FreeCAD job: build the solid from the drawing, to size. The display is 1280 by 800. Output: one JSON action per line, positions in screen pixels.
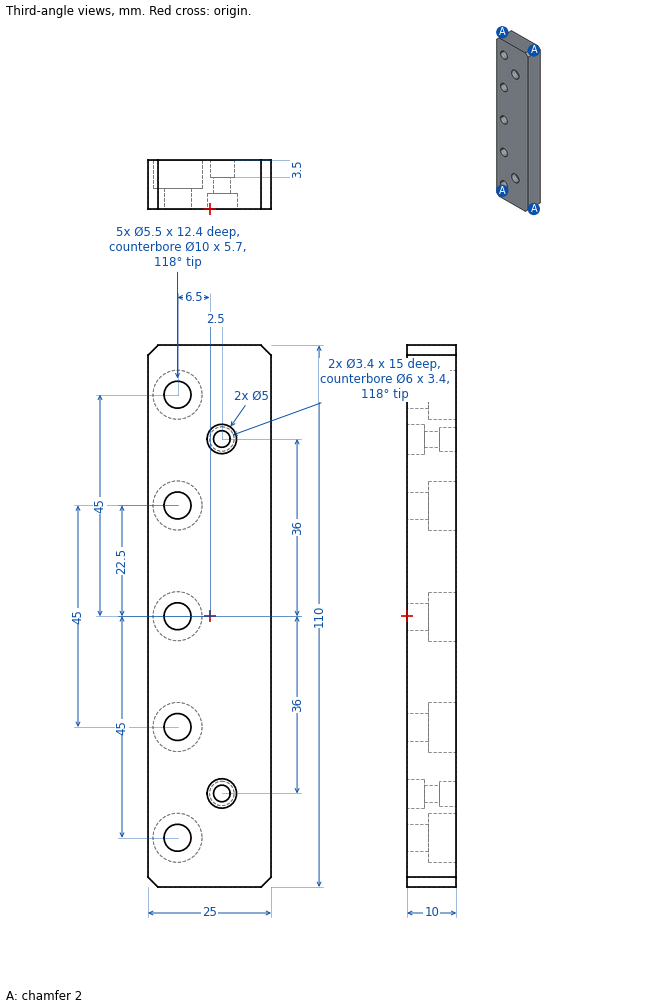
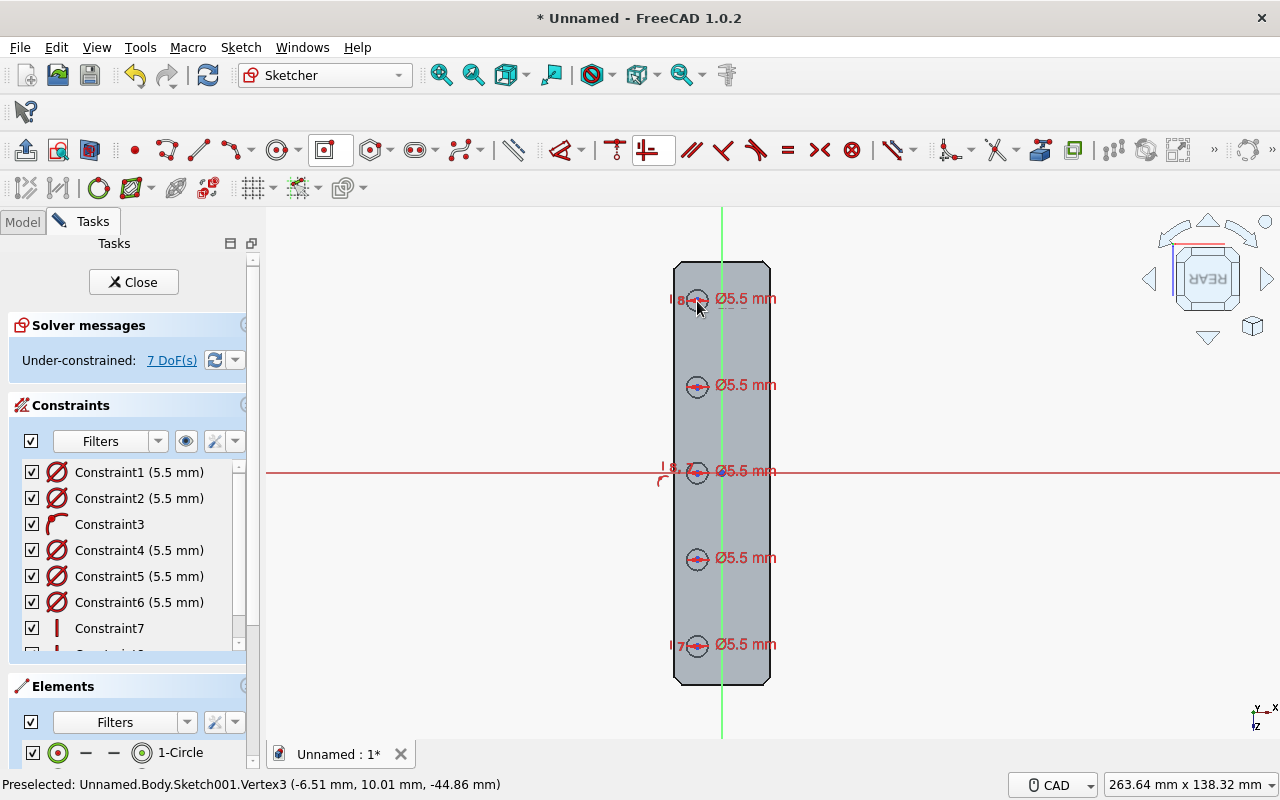
{"action": "left_click", "coordinate": [697, 646]}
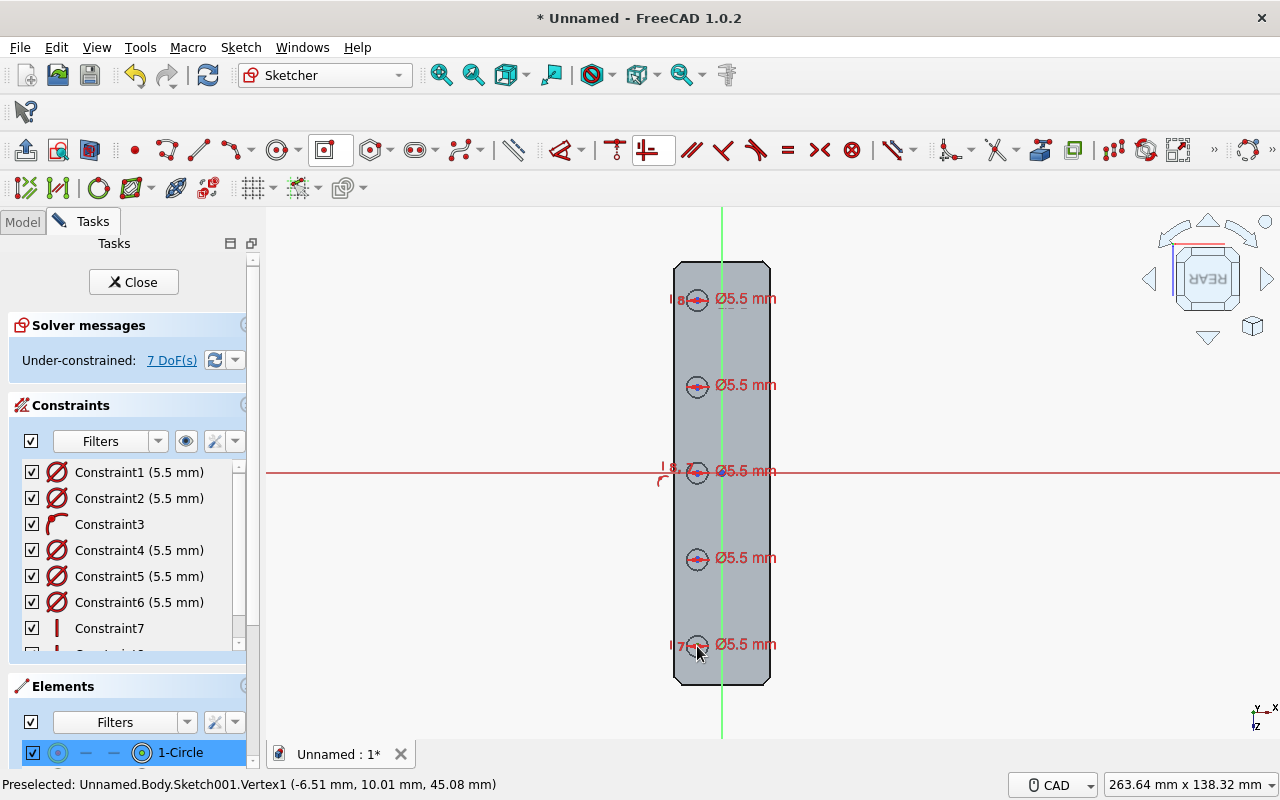
{"action": "left_click", "coordinate": [697, 560]}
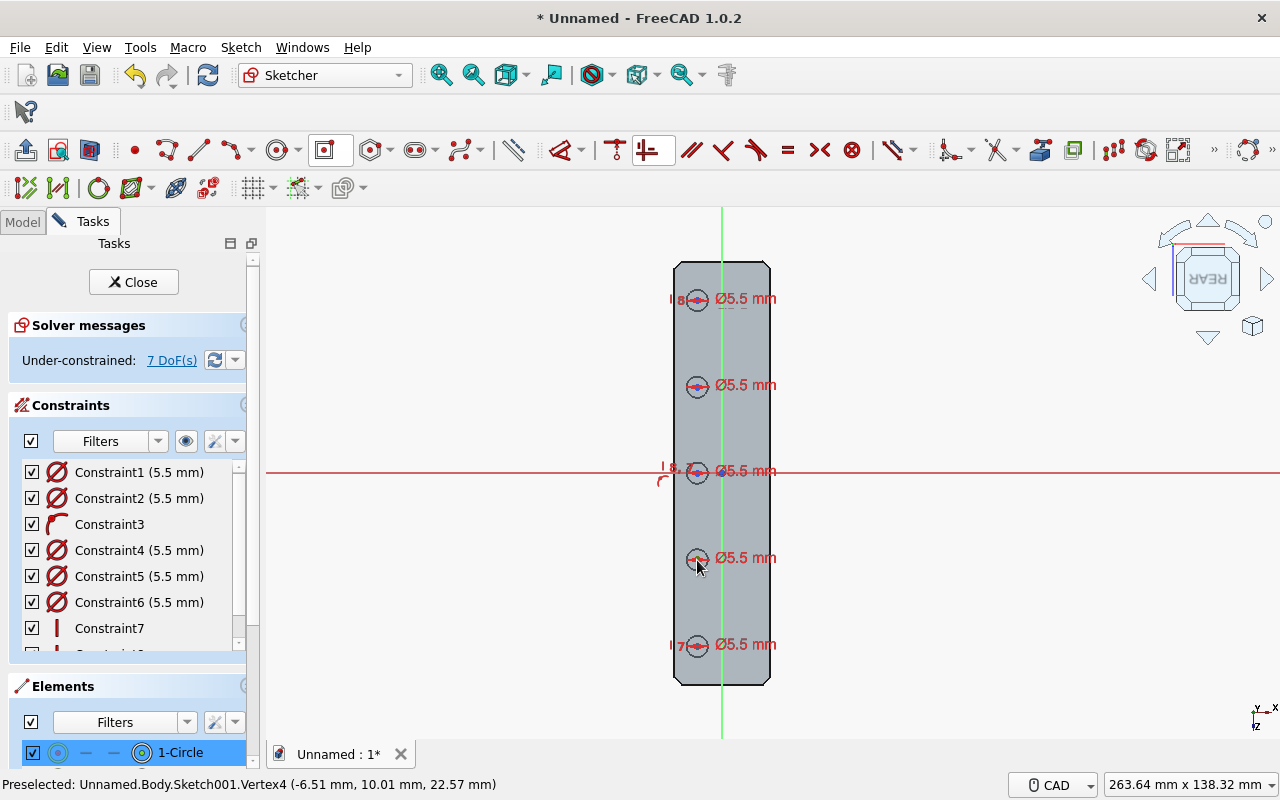
{"action": "key", "text": "v"}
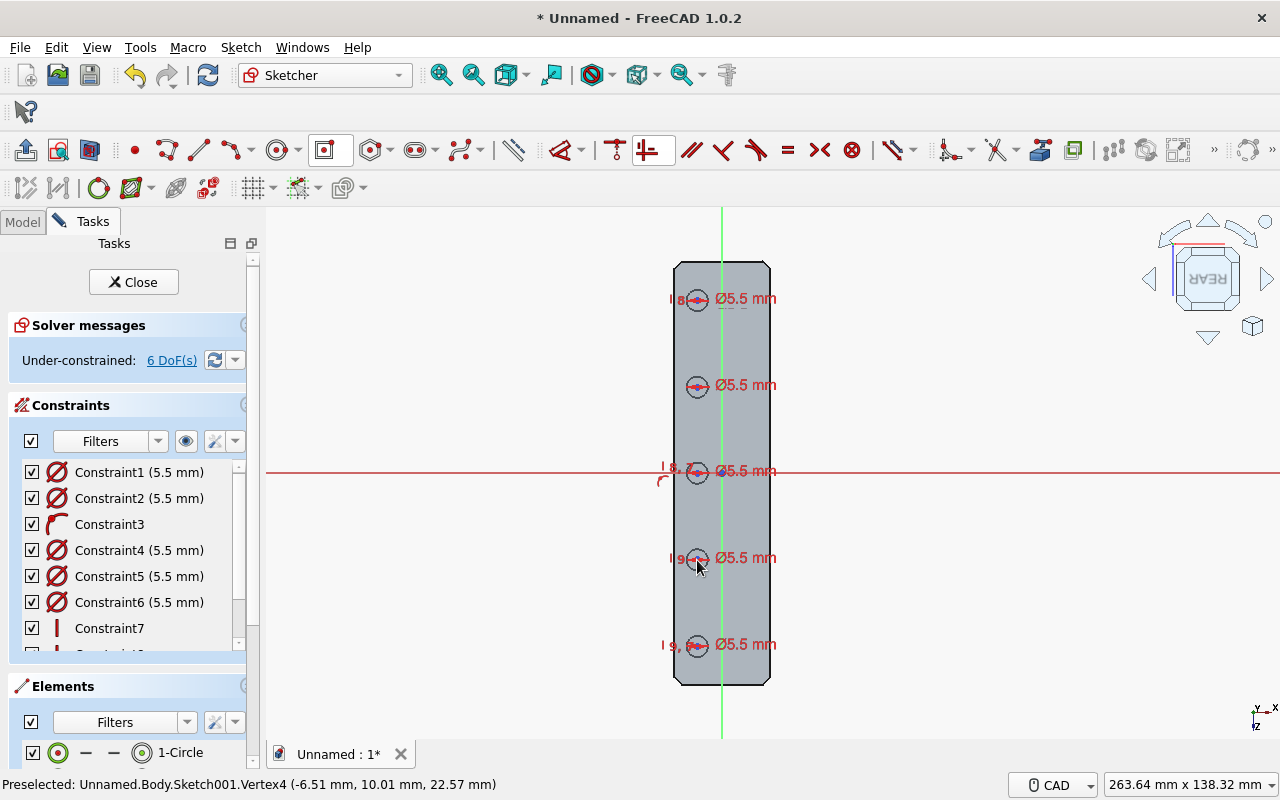
{"action": "left_click", "coordinate": [697, 473]}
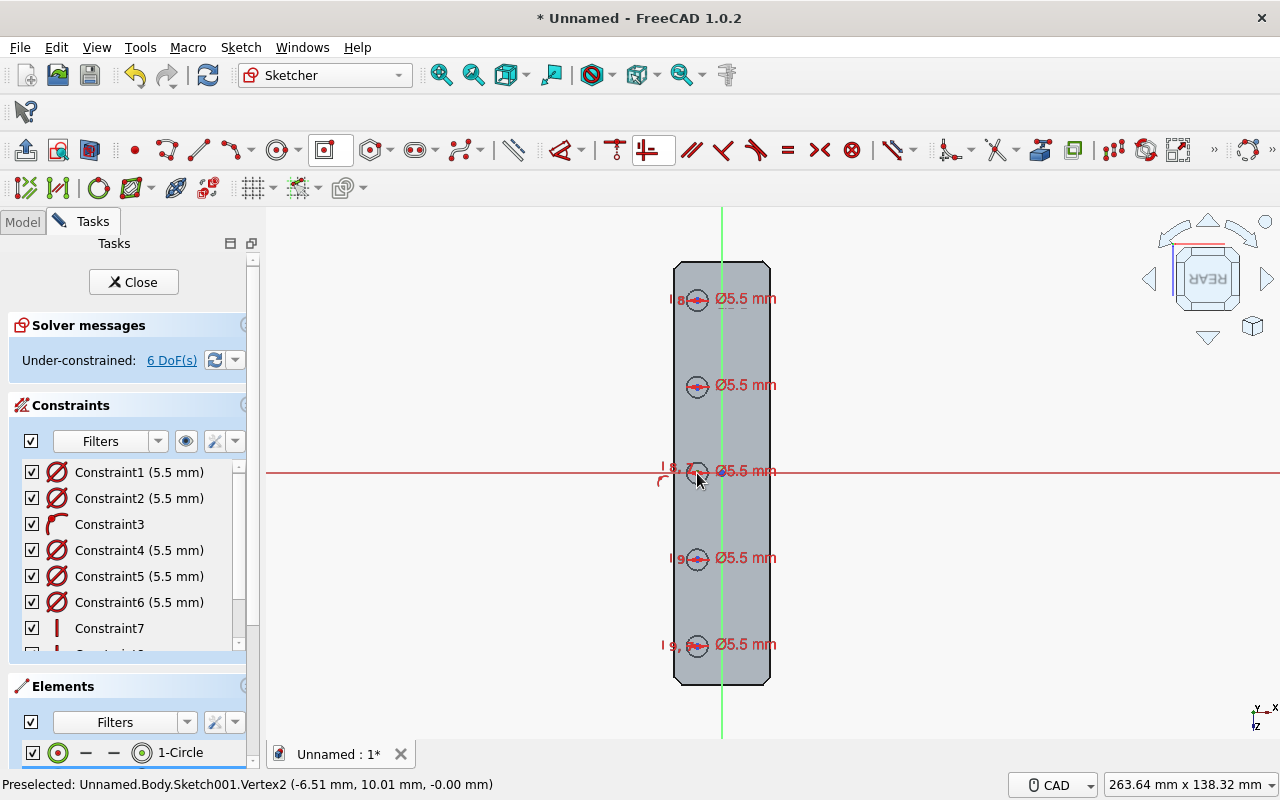
{"action": "left_click", "coordinate": [697, 387]}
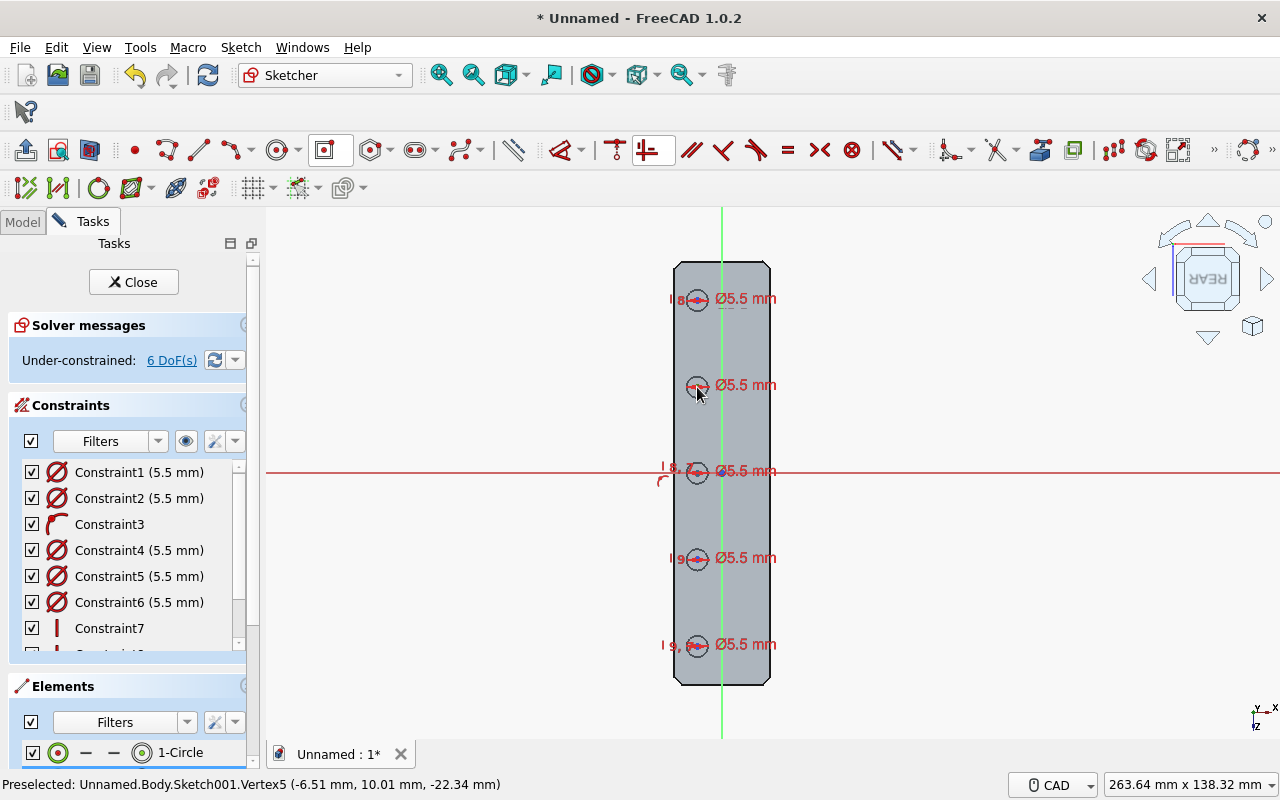
{"action": "left_click", "coordinate": [670, 150]}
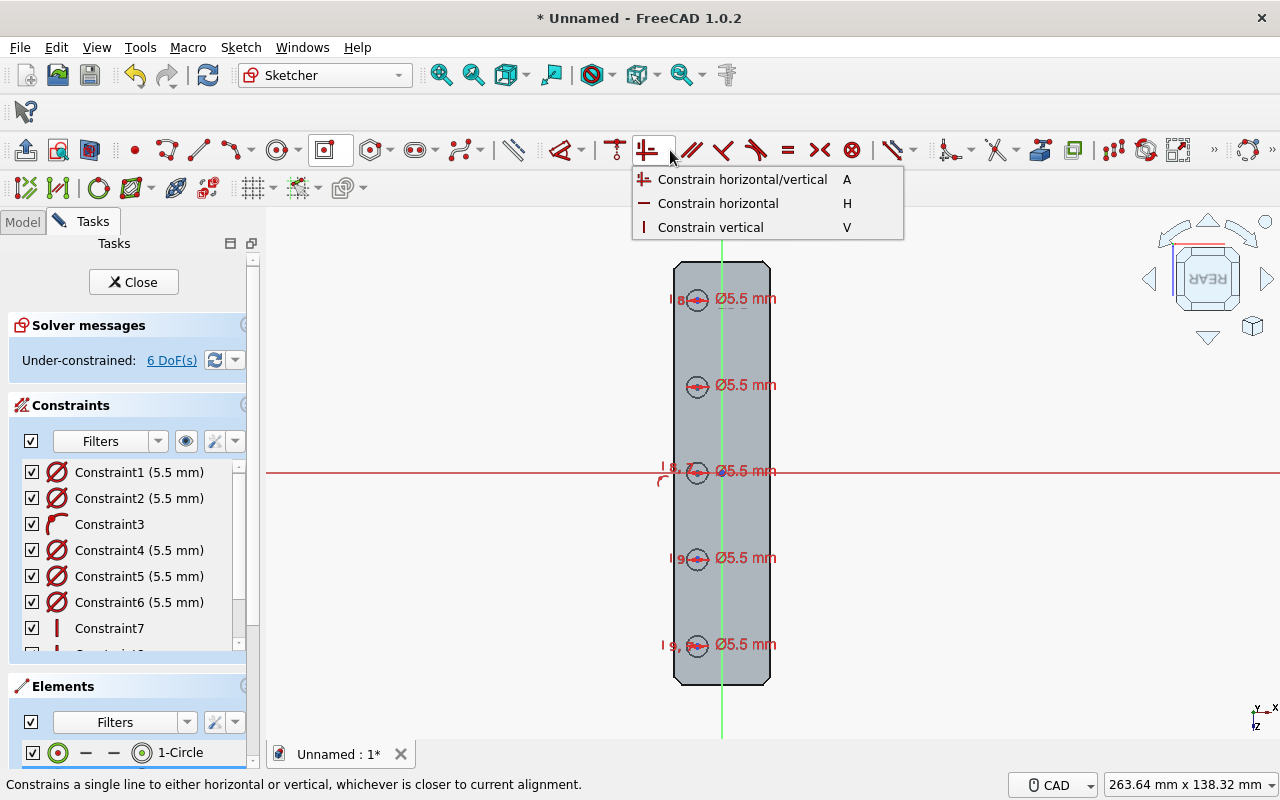
{"action": "left_click", "coordinate": [768, 227]}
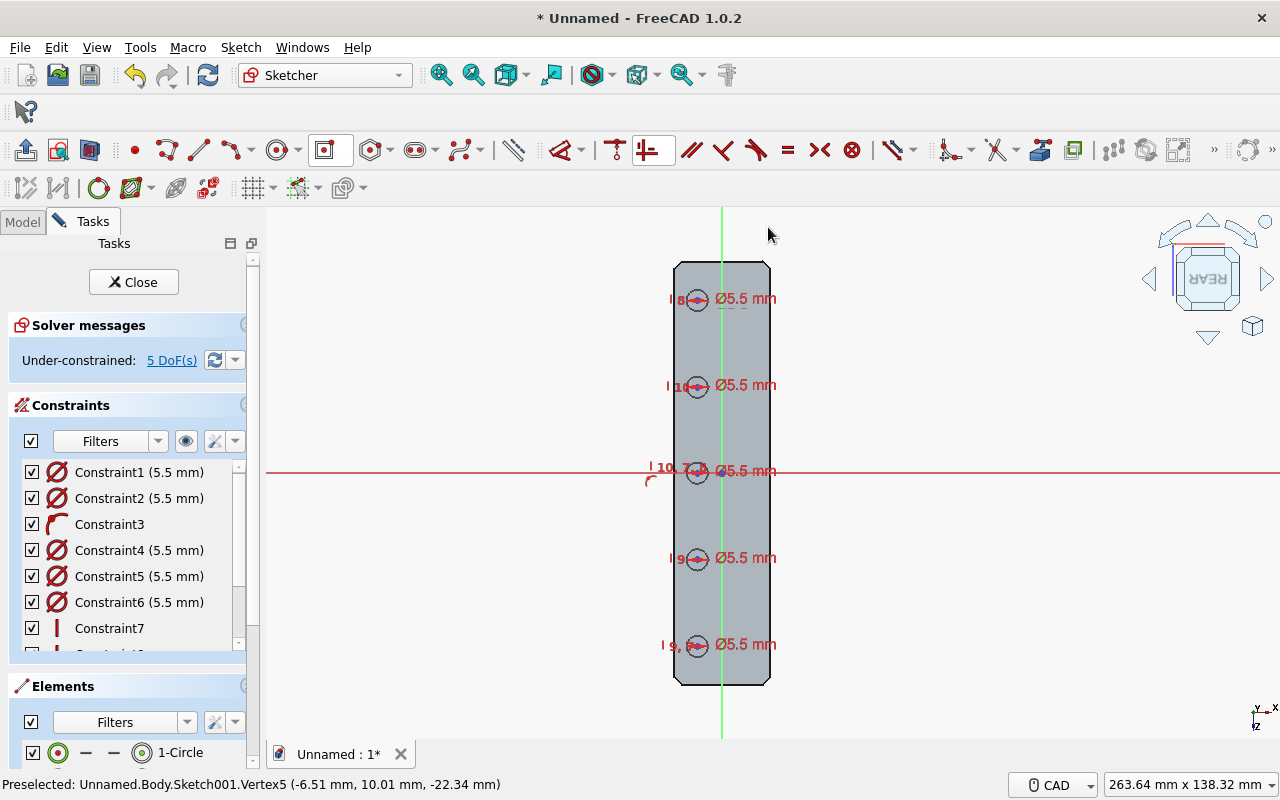
{"action": "left_click", "coordinate": [560, 150]}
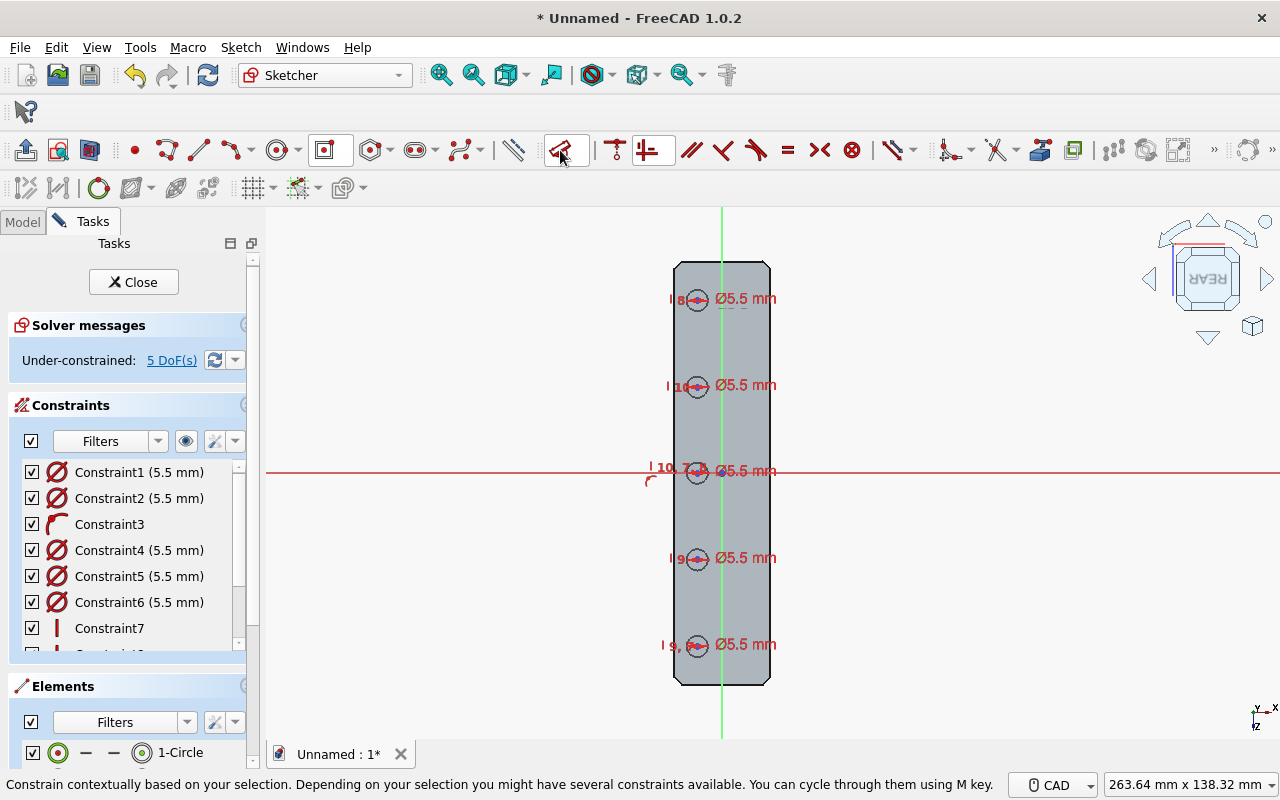
{"action": "left_click", "coordinate": [697, 646]}
{"action": "left_click", "coordinate": [756, 560]}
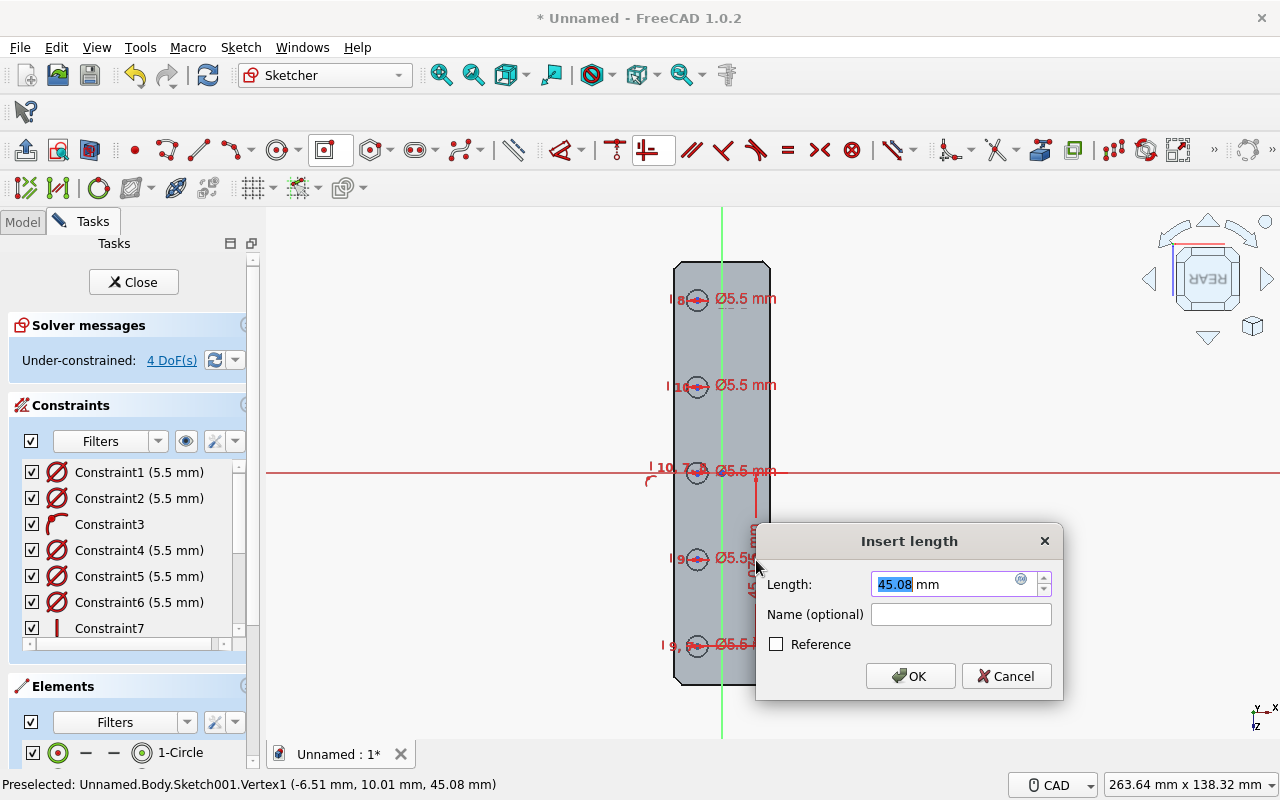
{"action": "type", "text": "45"}
{"action": "key", "text": "Return"}